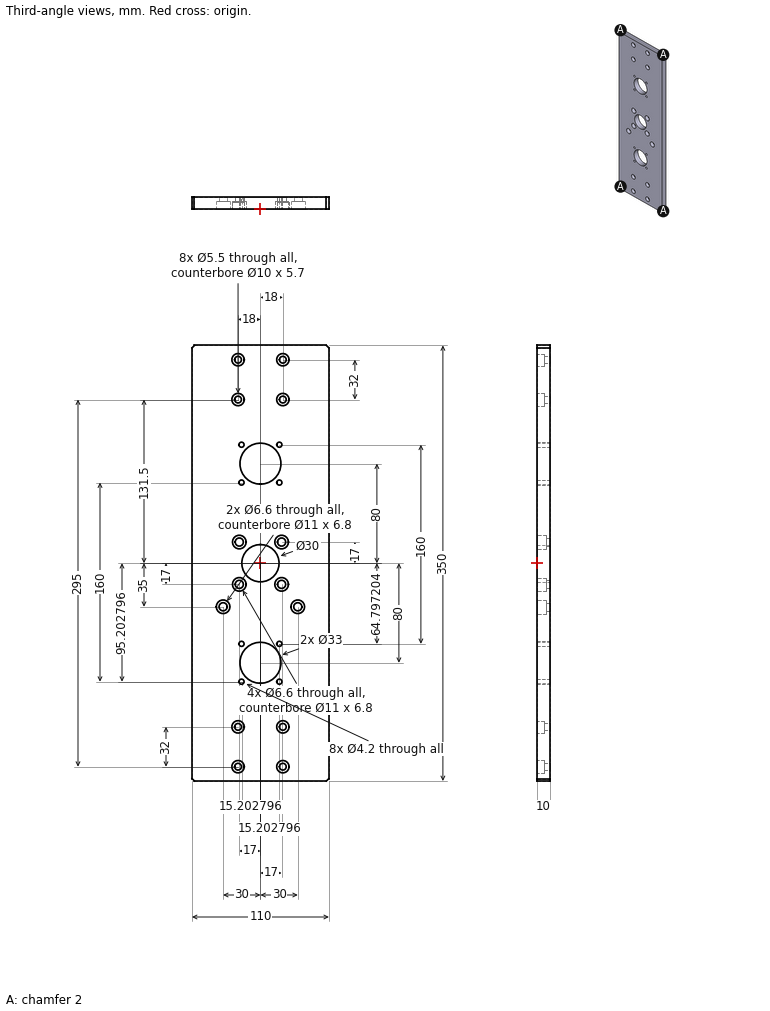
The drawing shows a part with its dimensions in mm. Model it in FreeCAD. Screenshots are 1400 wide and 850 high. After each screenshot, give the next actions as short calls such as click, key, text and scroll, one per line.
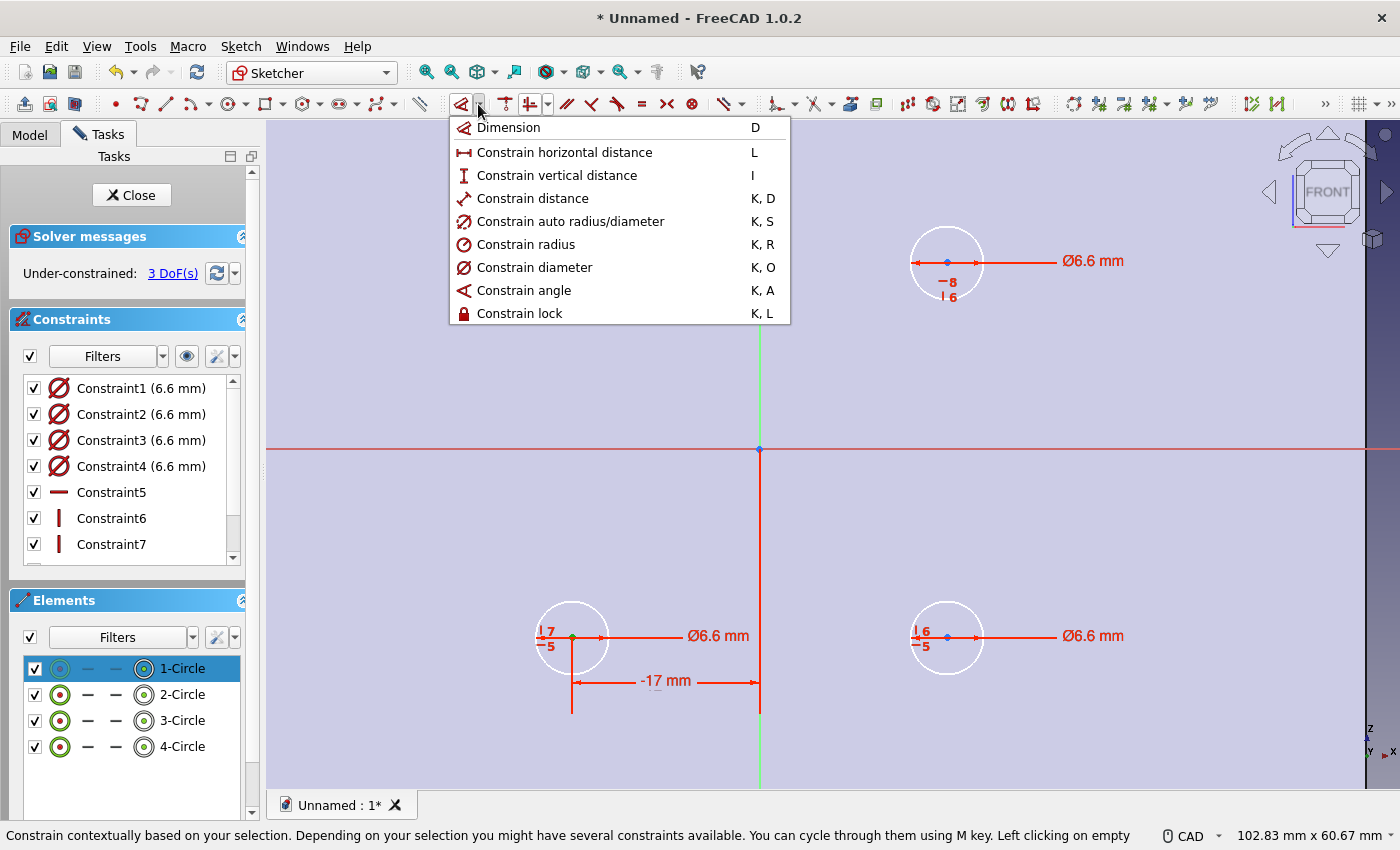
click(620, 176)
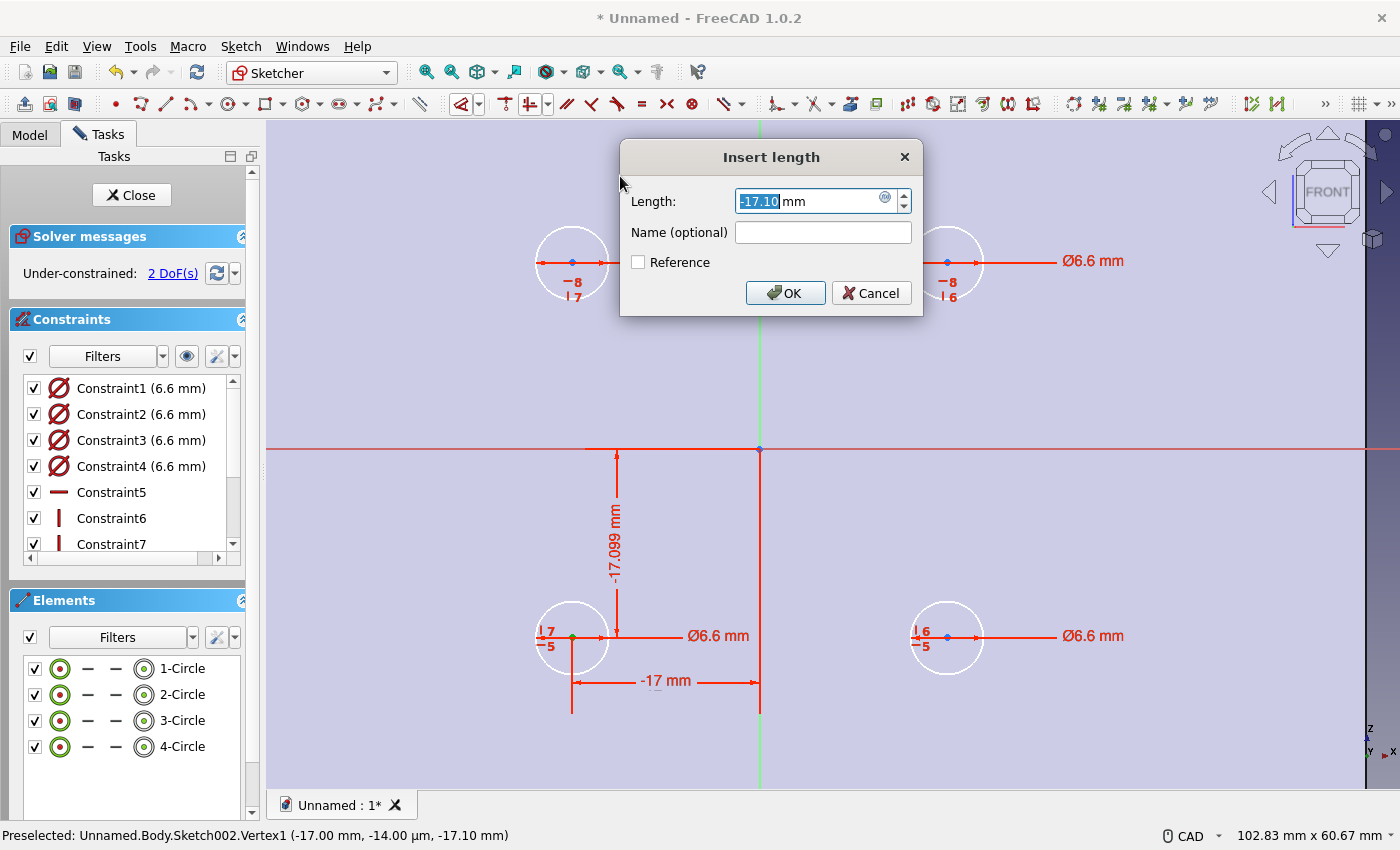
text(-17)
key(Return)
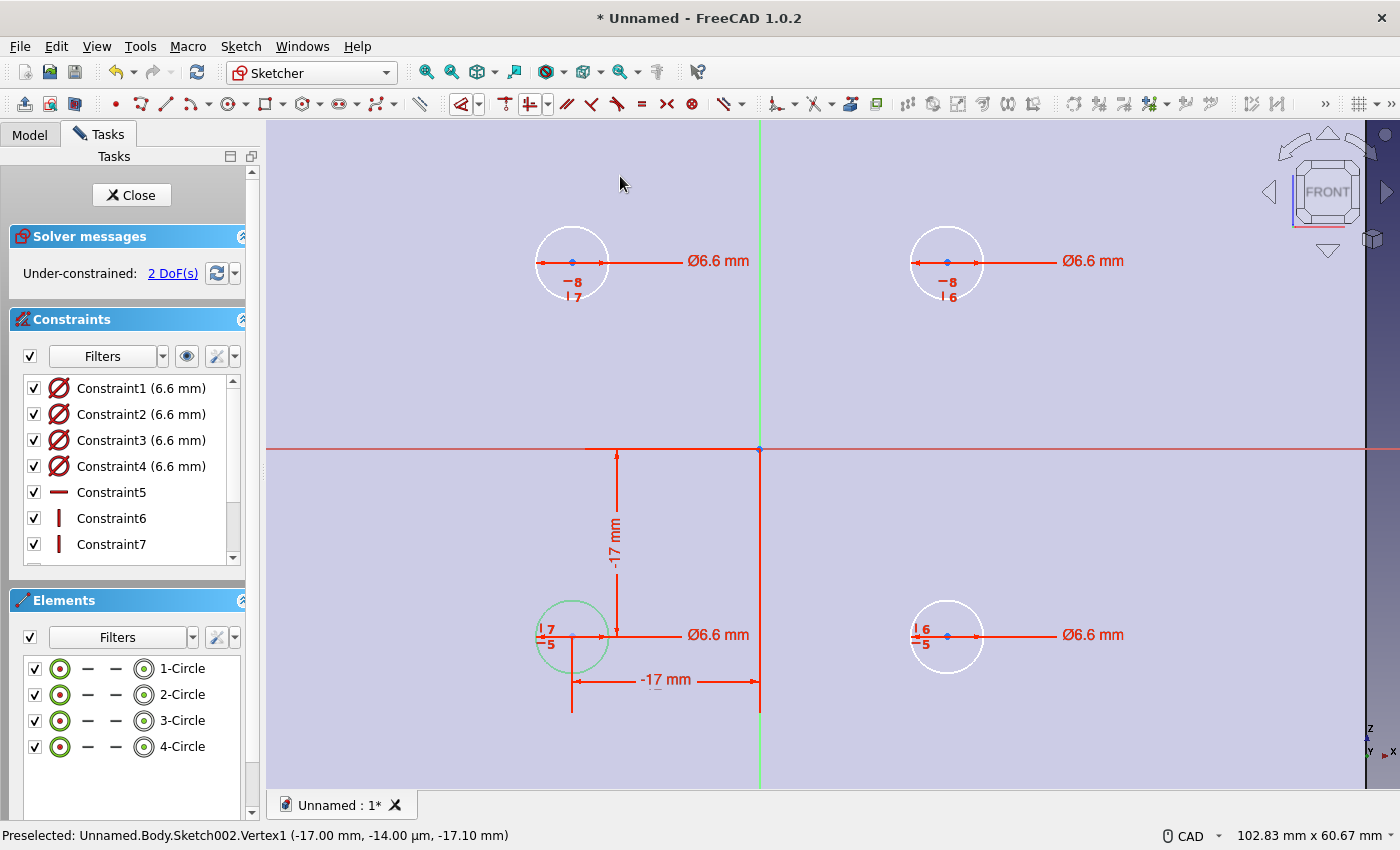
click(947, 637)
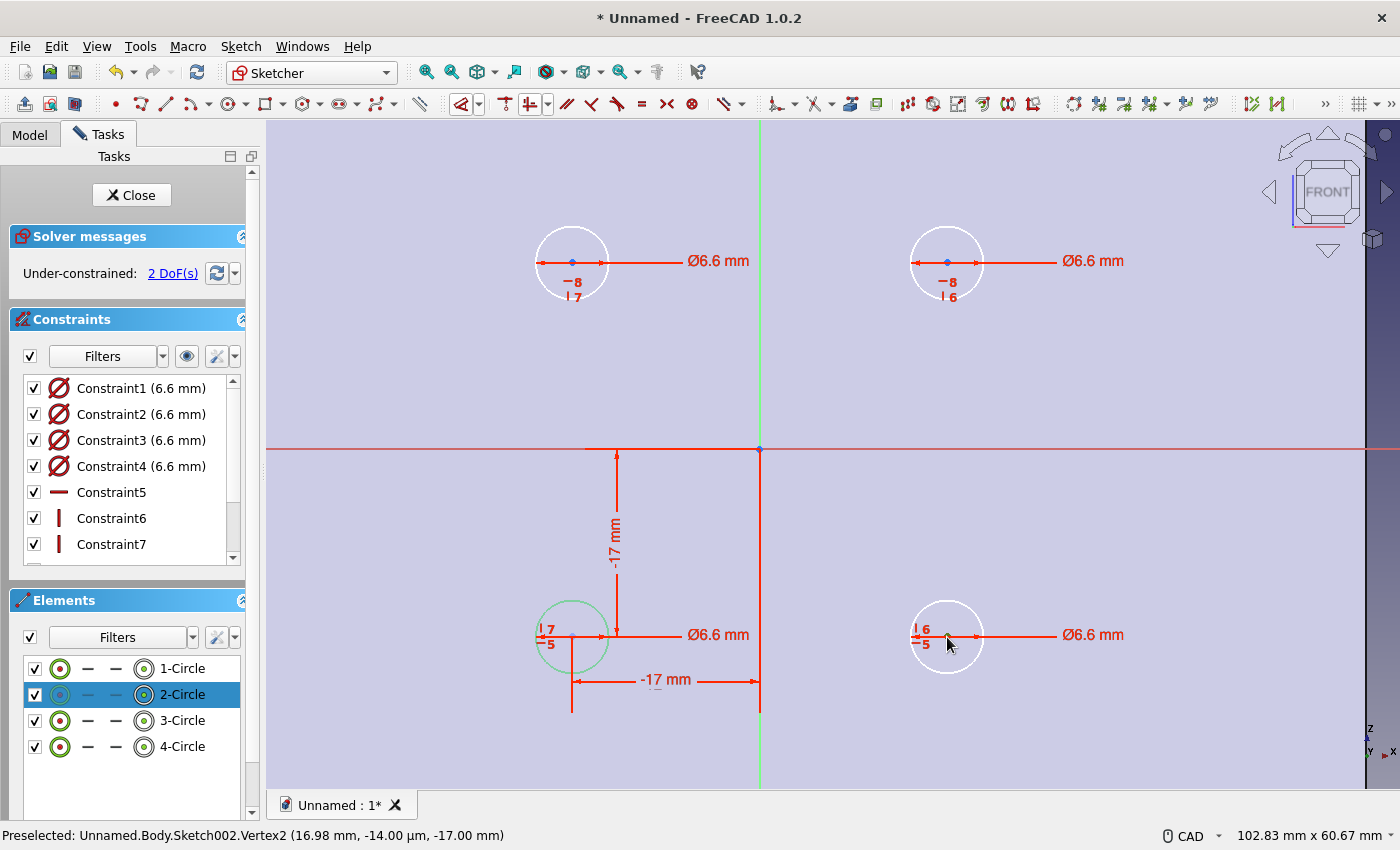
key(l)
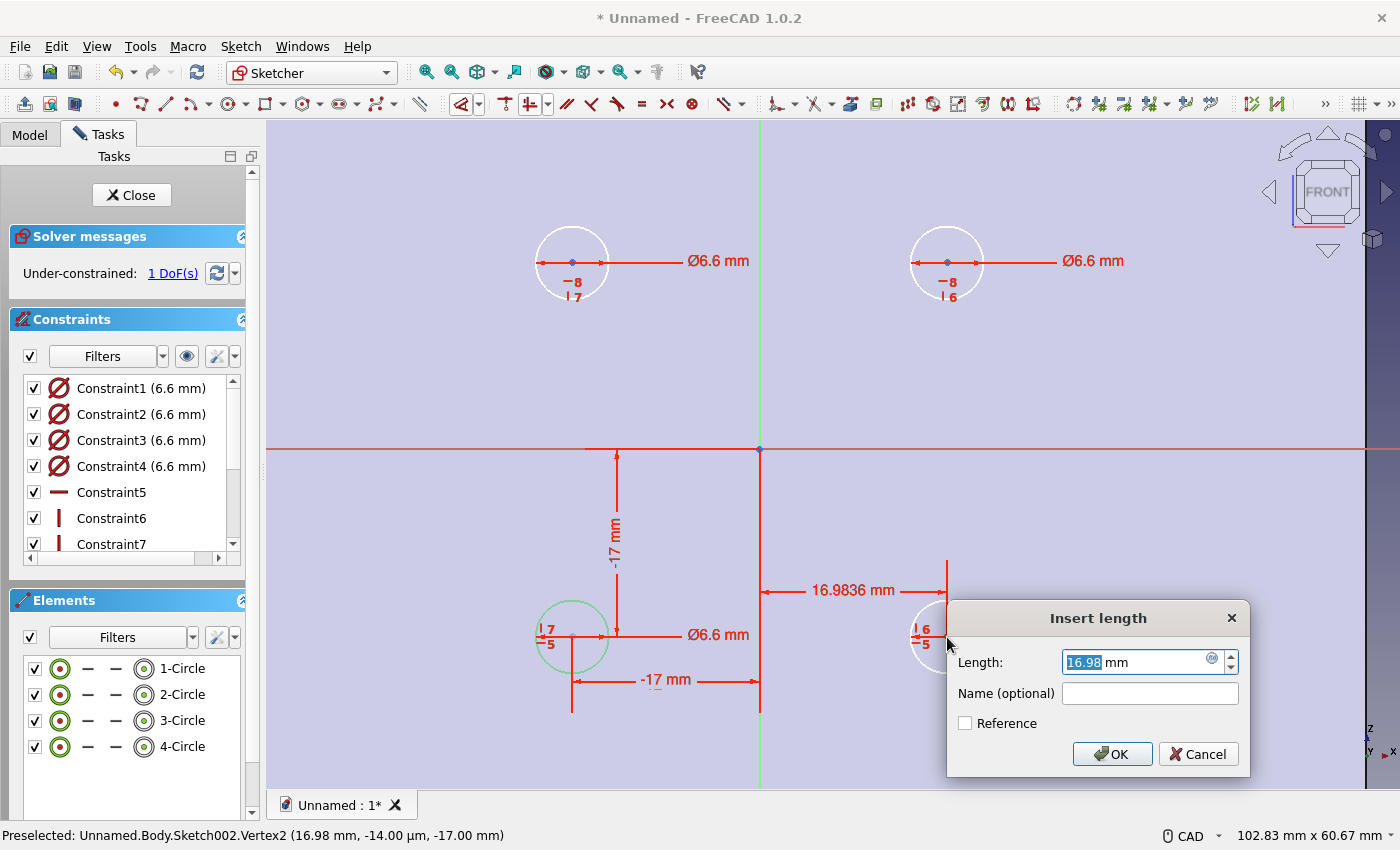
text(17)
key(Return)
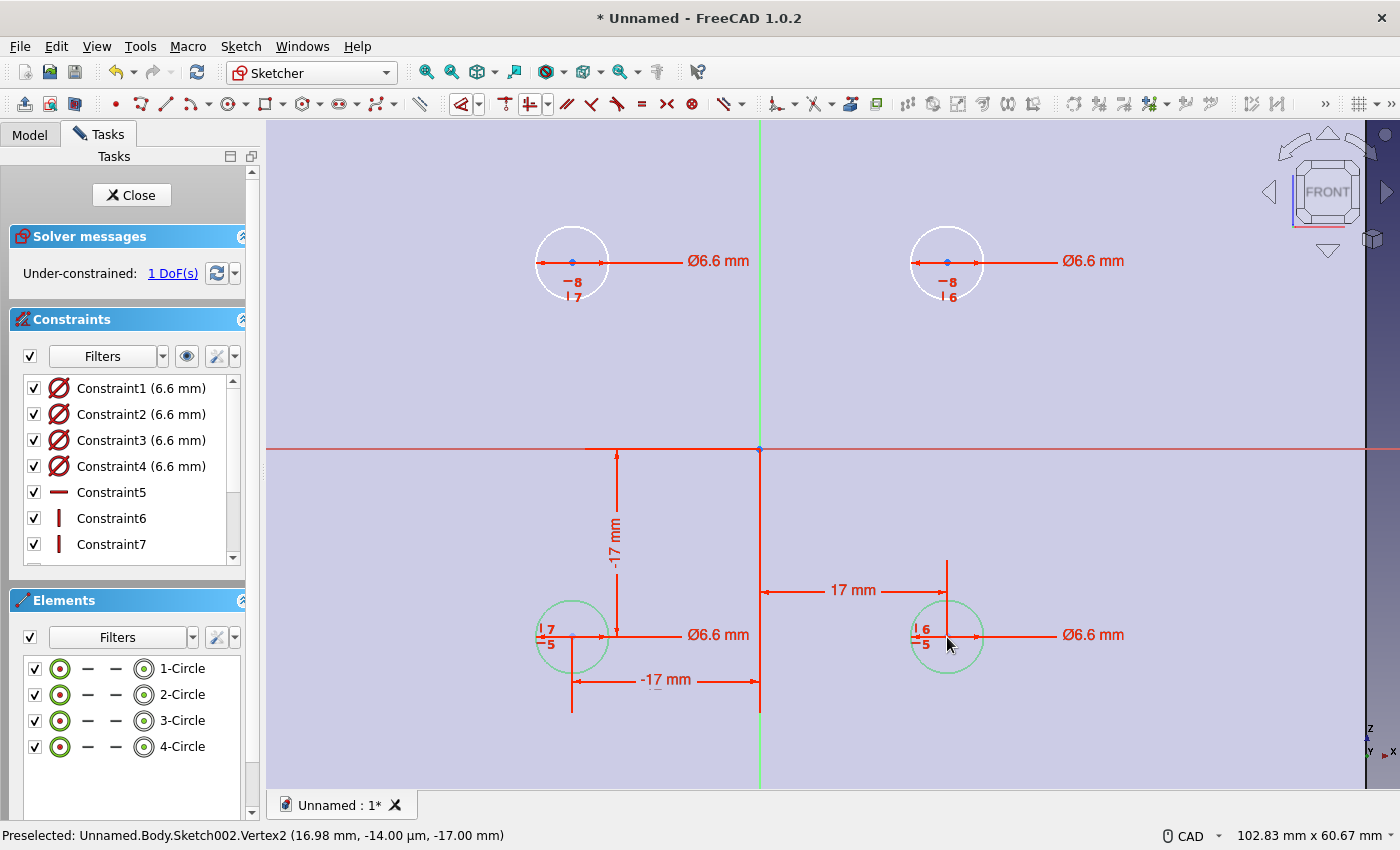
click(947, 263)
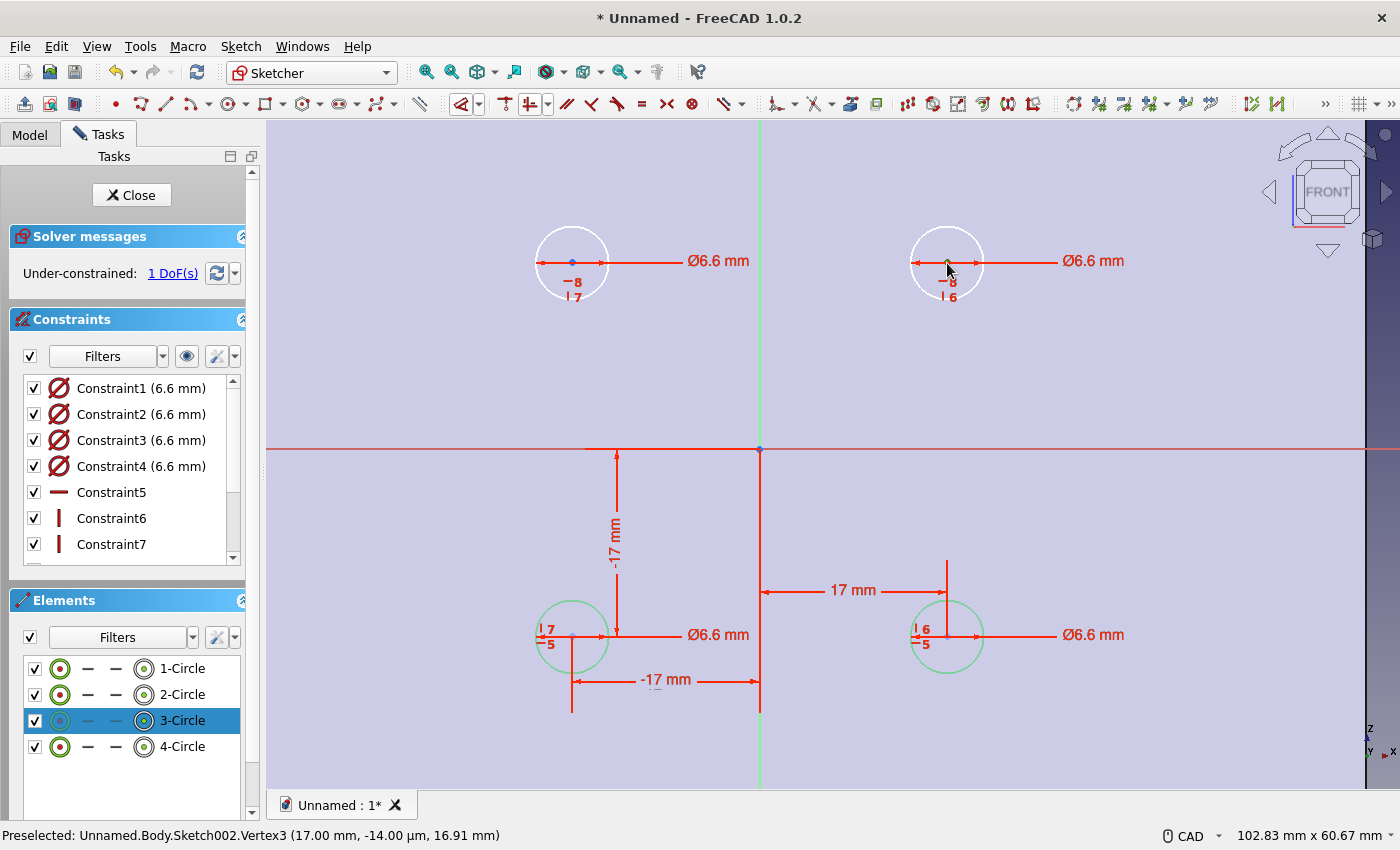
key(i)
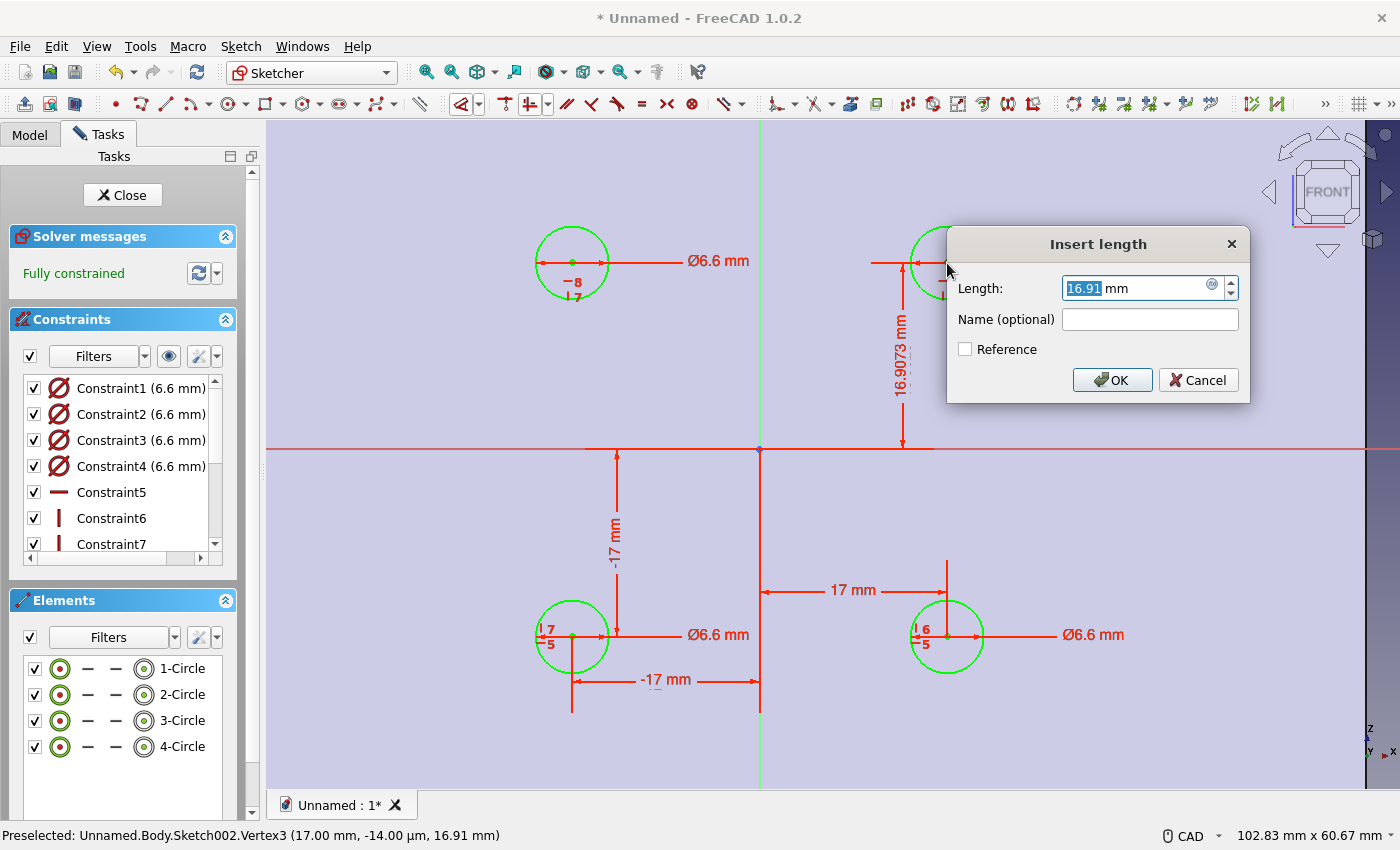
text(17)
key(Return)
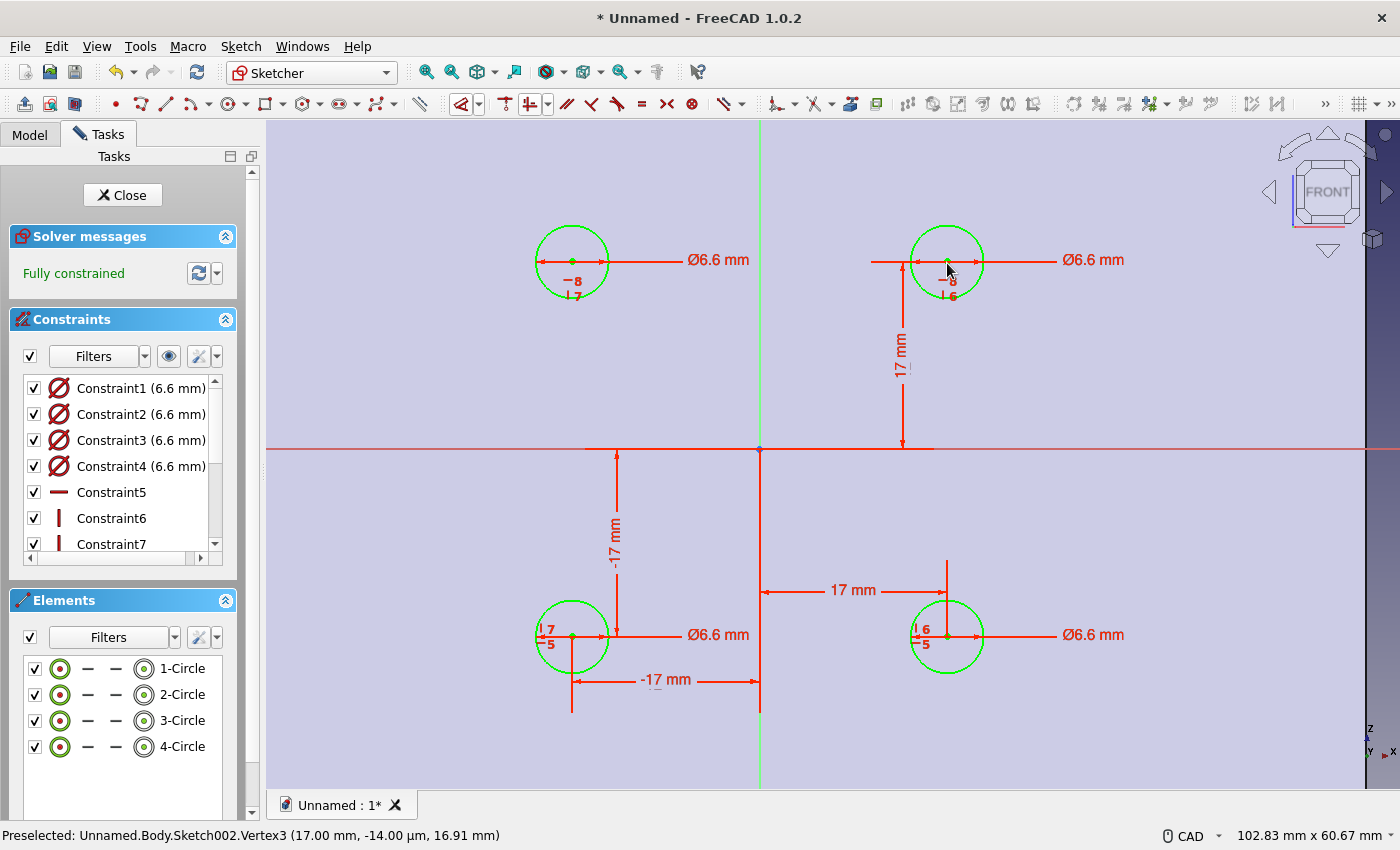
click(123, 195)